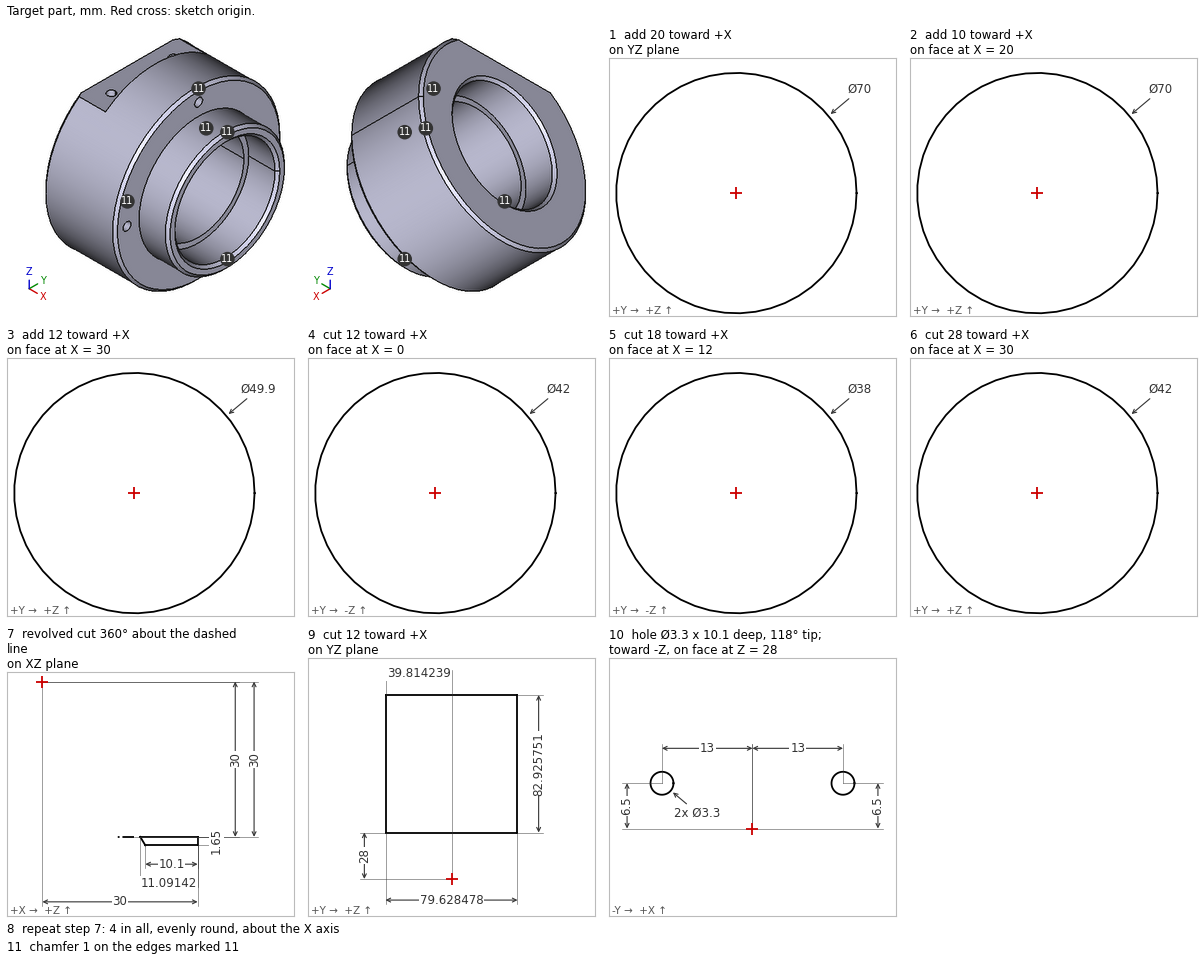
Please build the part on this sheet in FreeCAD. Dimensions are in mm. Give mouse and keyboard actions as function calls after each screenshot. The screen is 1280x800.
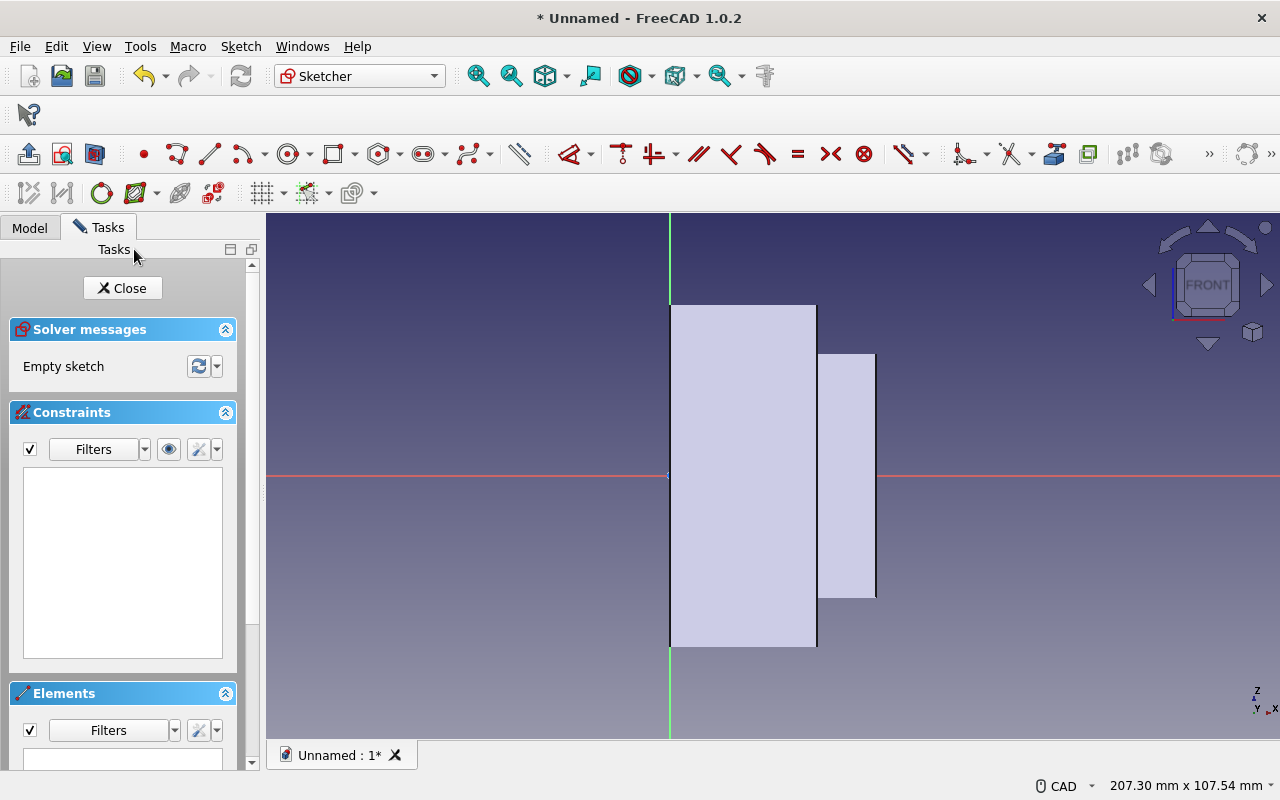
key(q)
key(s)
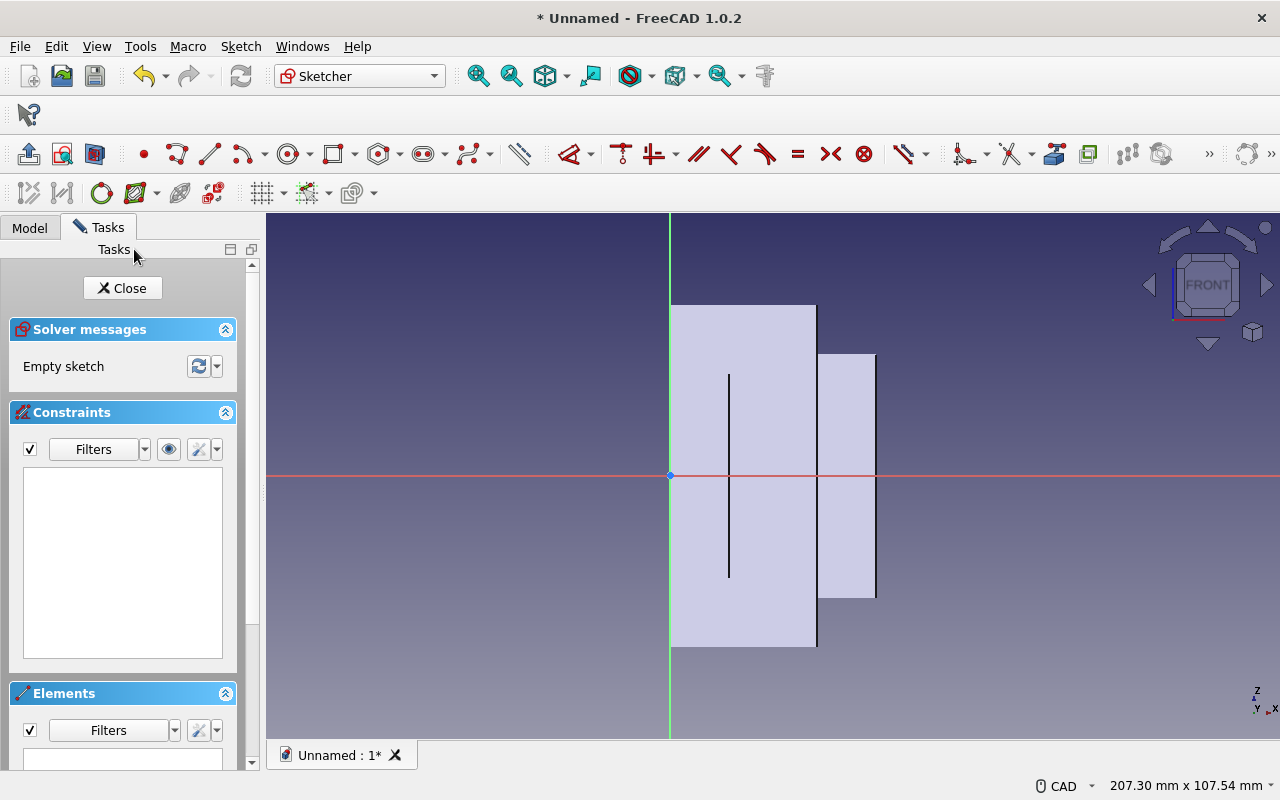
scroll(776, 617, up, 4)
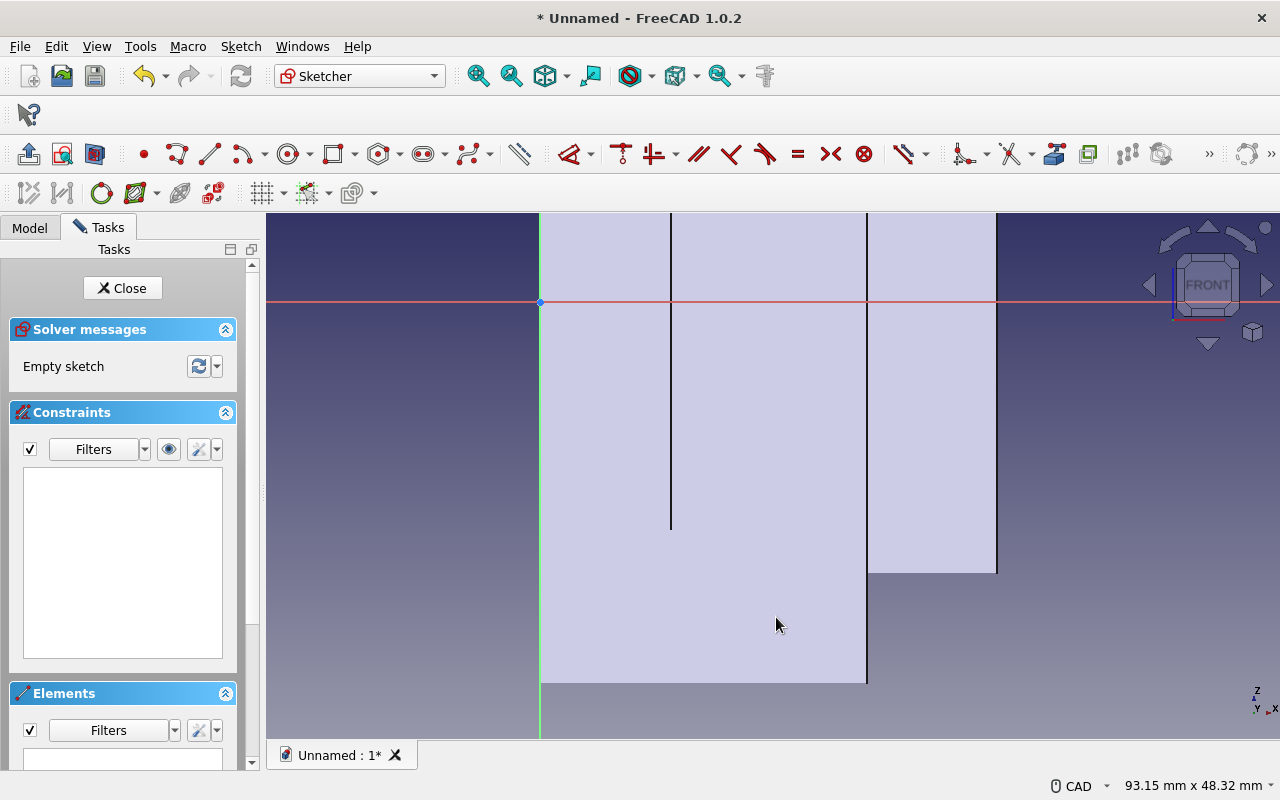
click(177, 154)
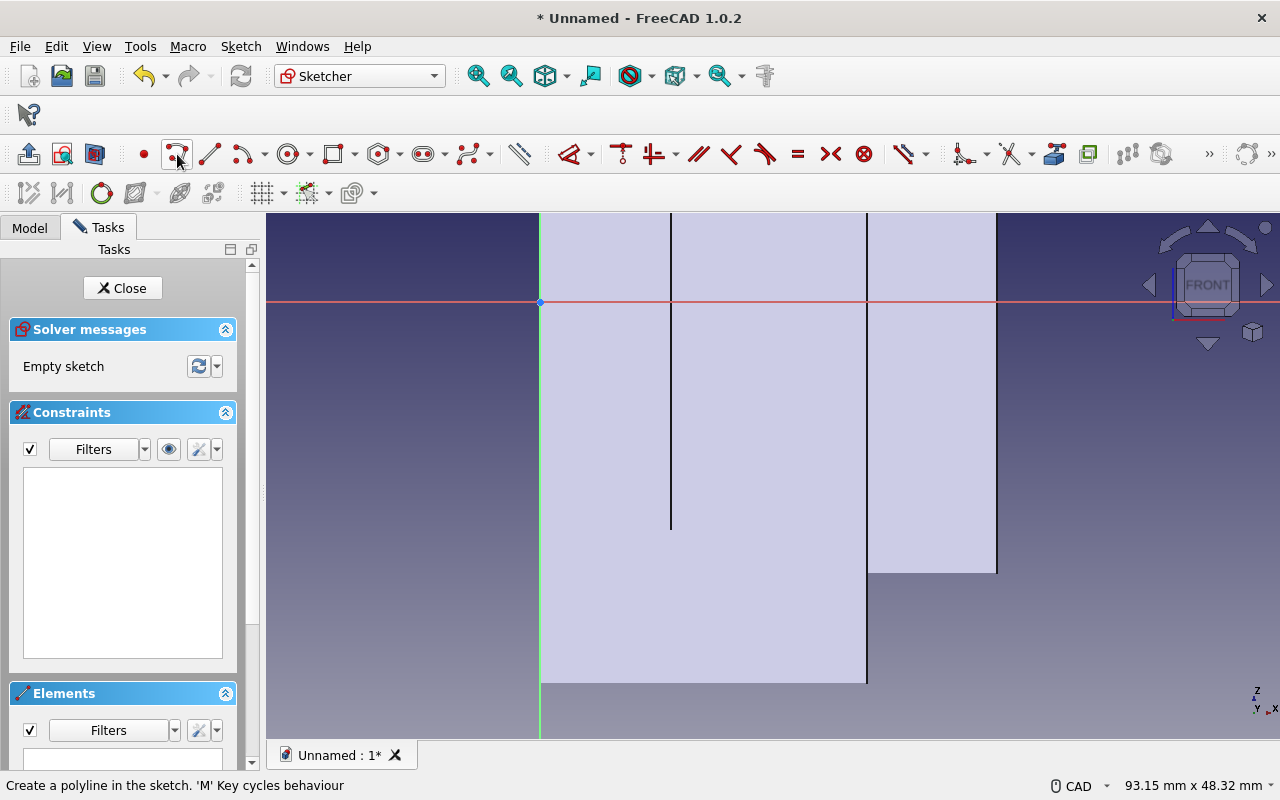
click(746, 629)
click(867, 629)
click(867, 647)
click(757, 647)
click(746, 630)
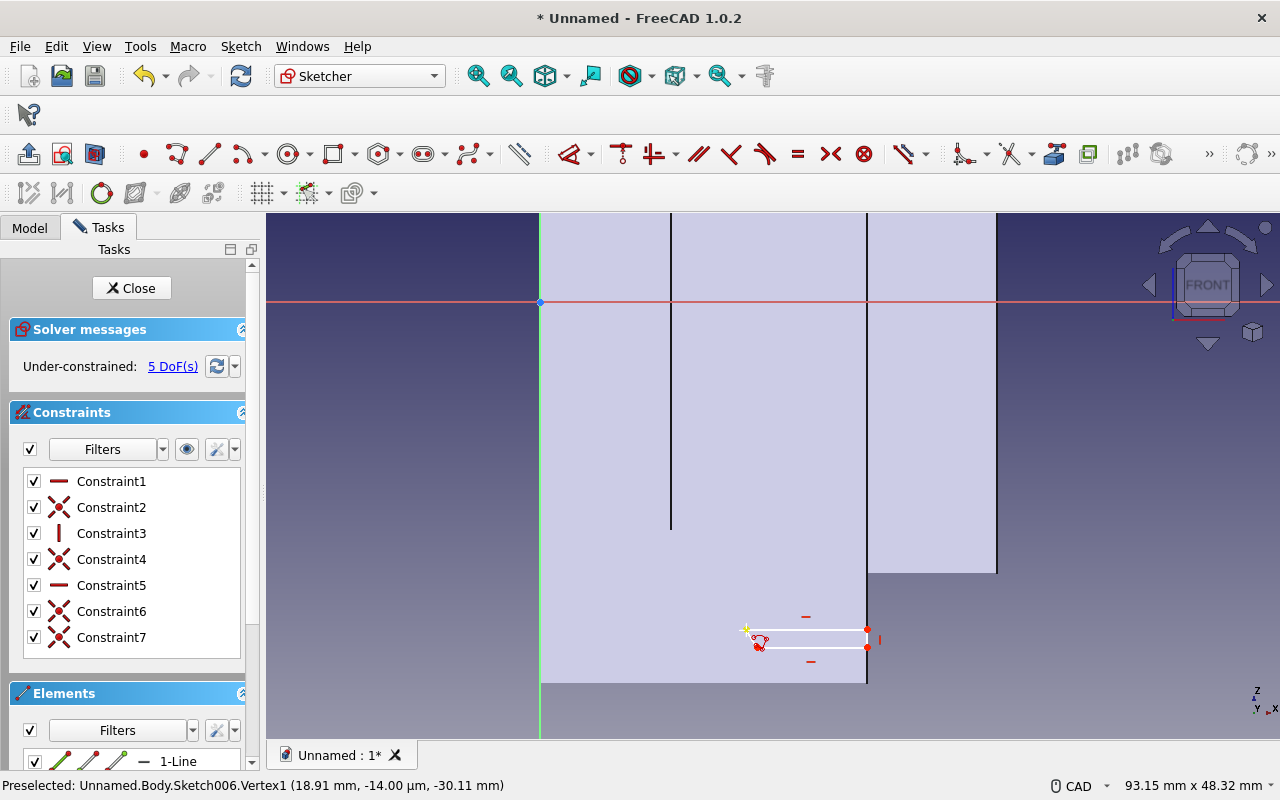
click(210, 154)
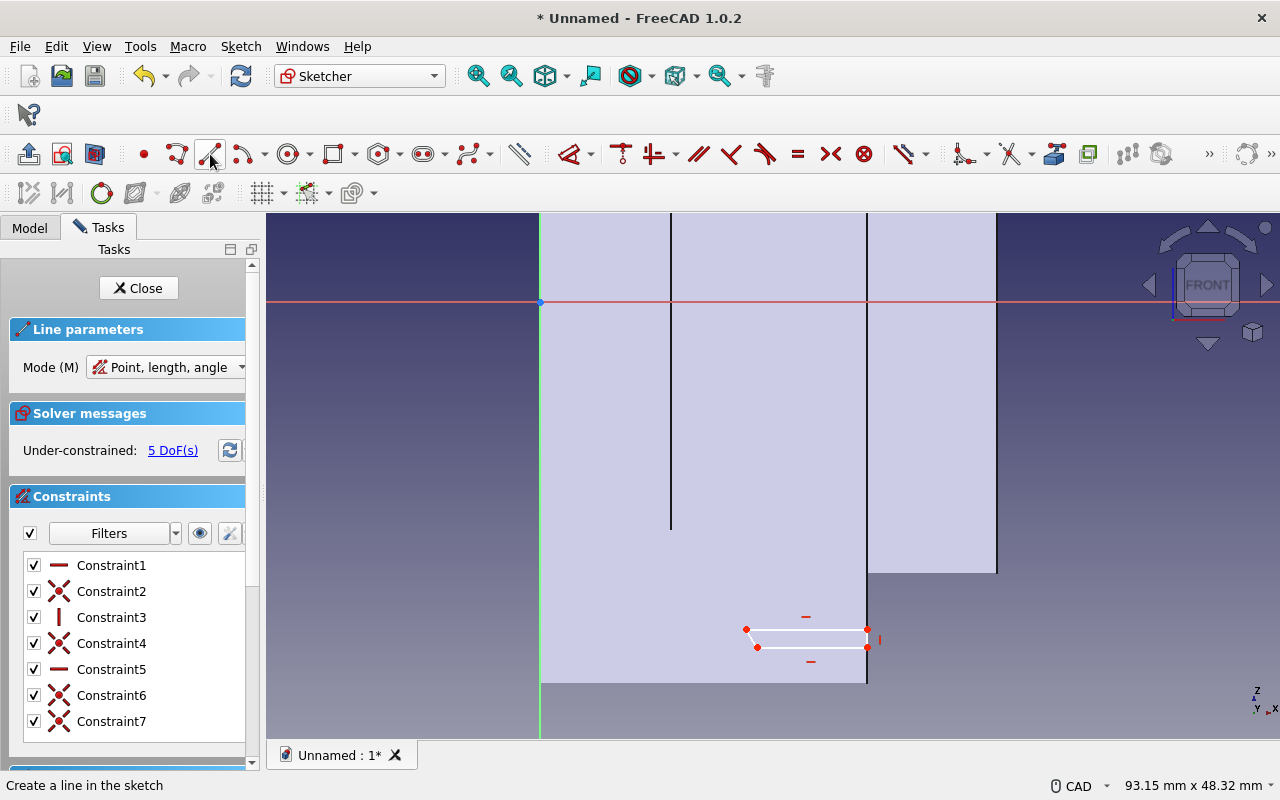
scroll(734, 629, up, 2)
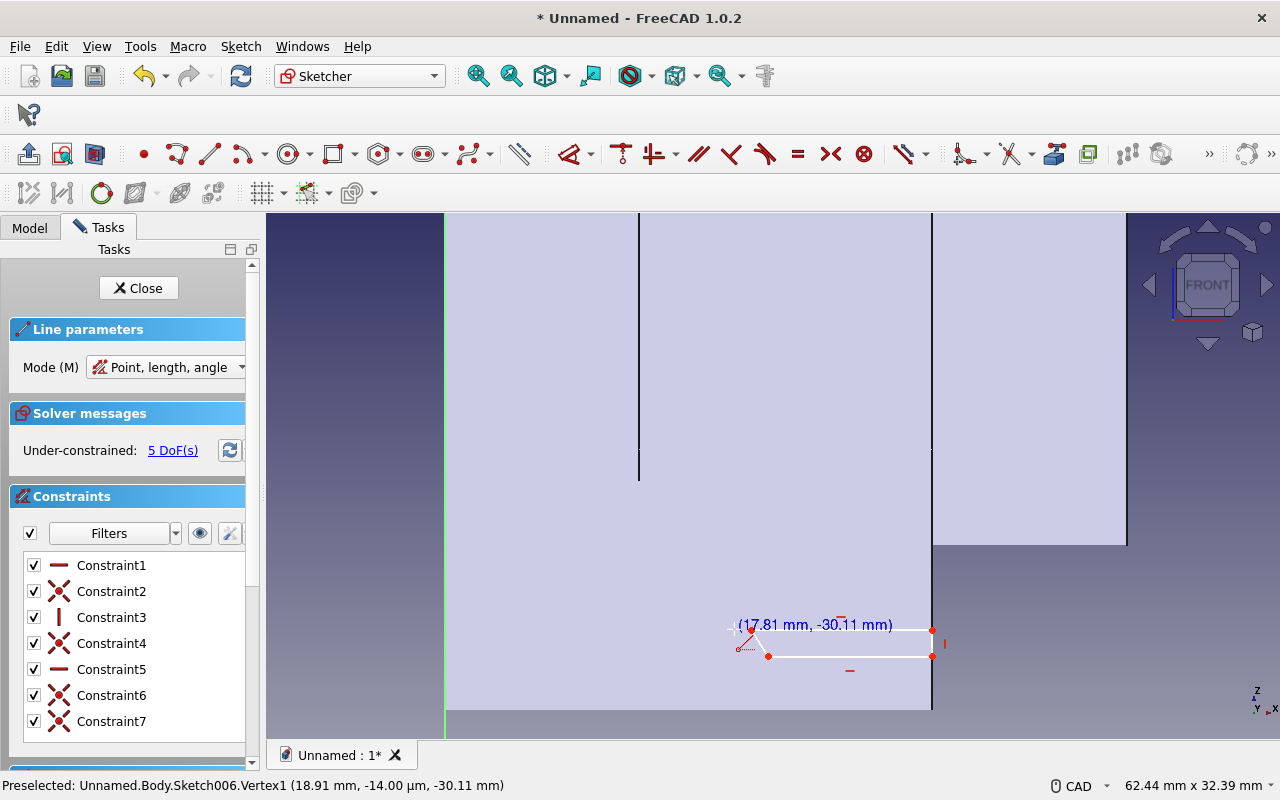
click(734, 628)
click(680, 628)
key(Escape)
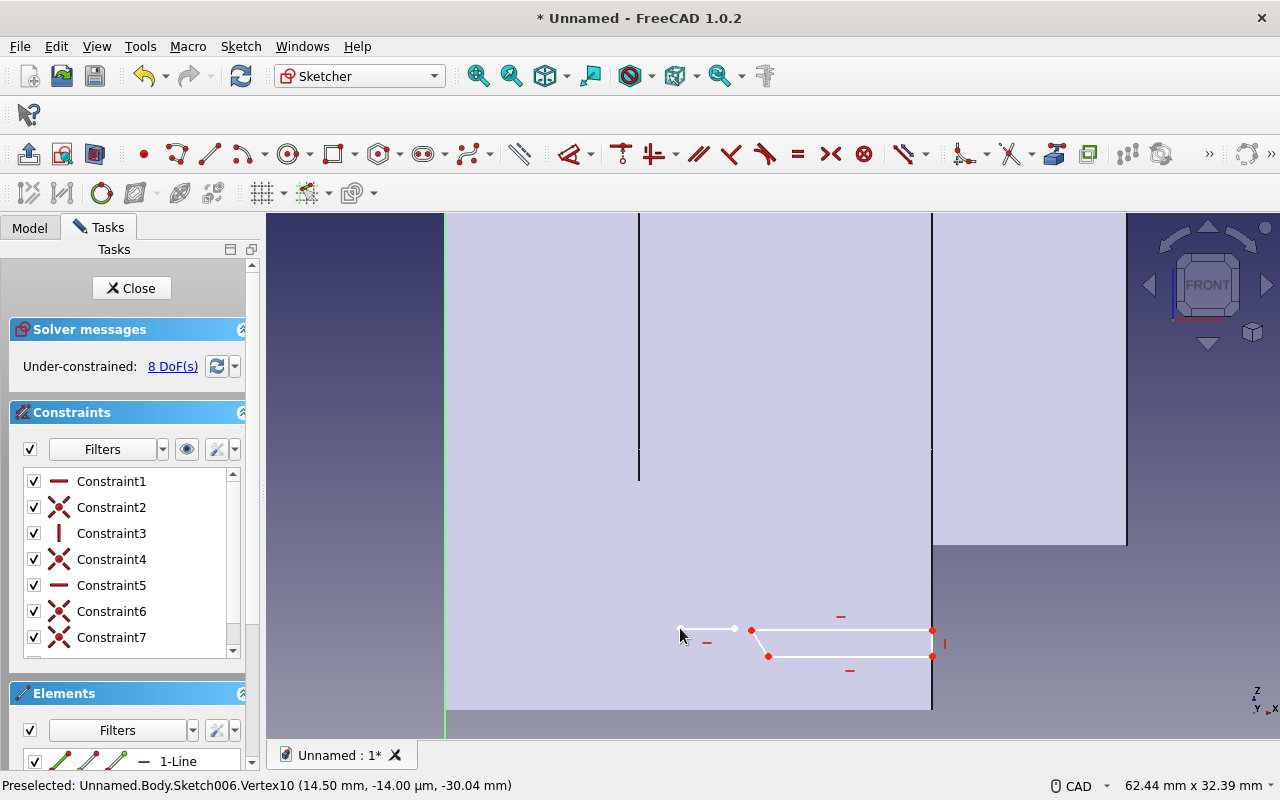
click(718, 629)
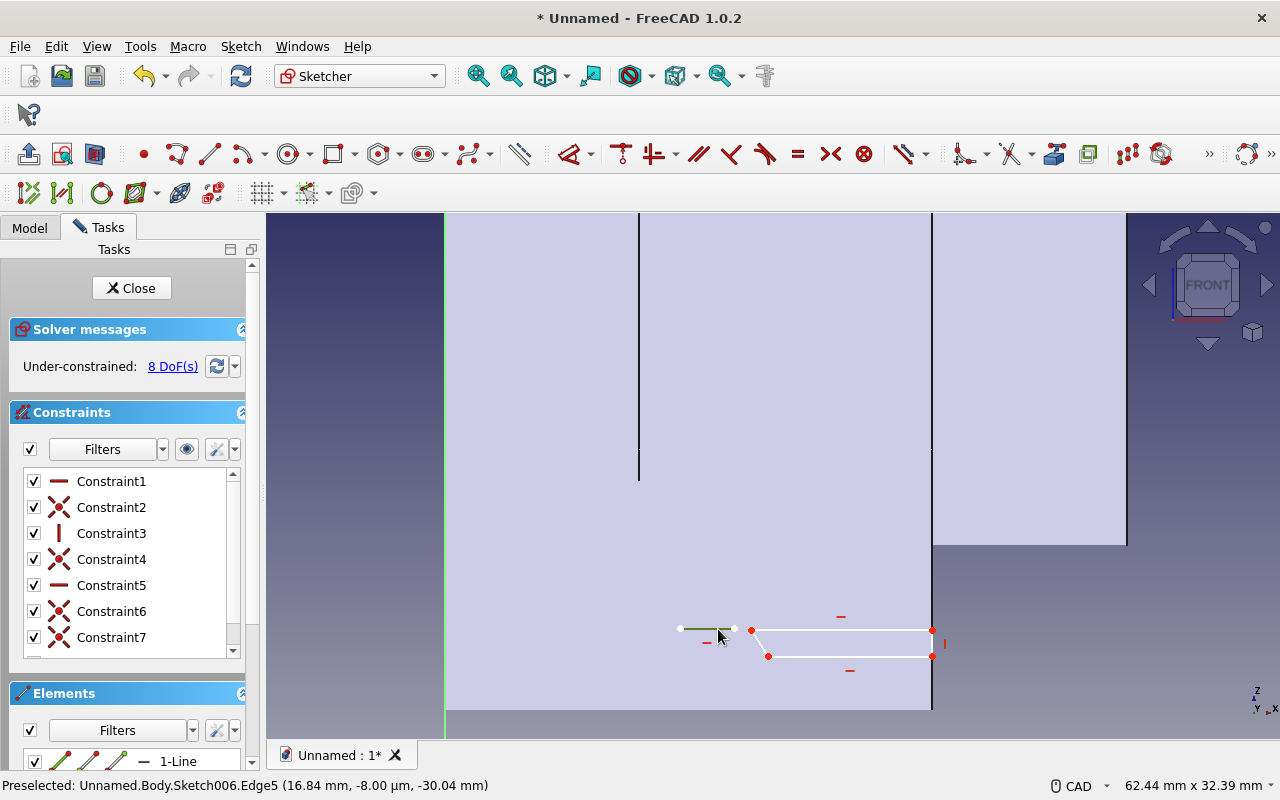
click(520, 154)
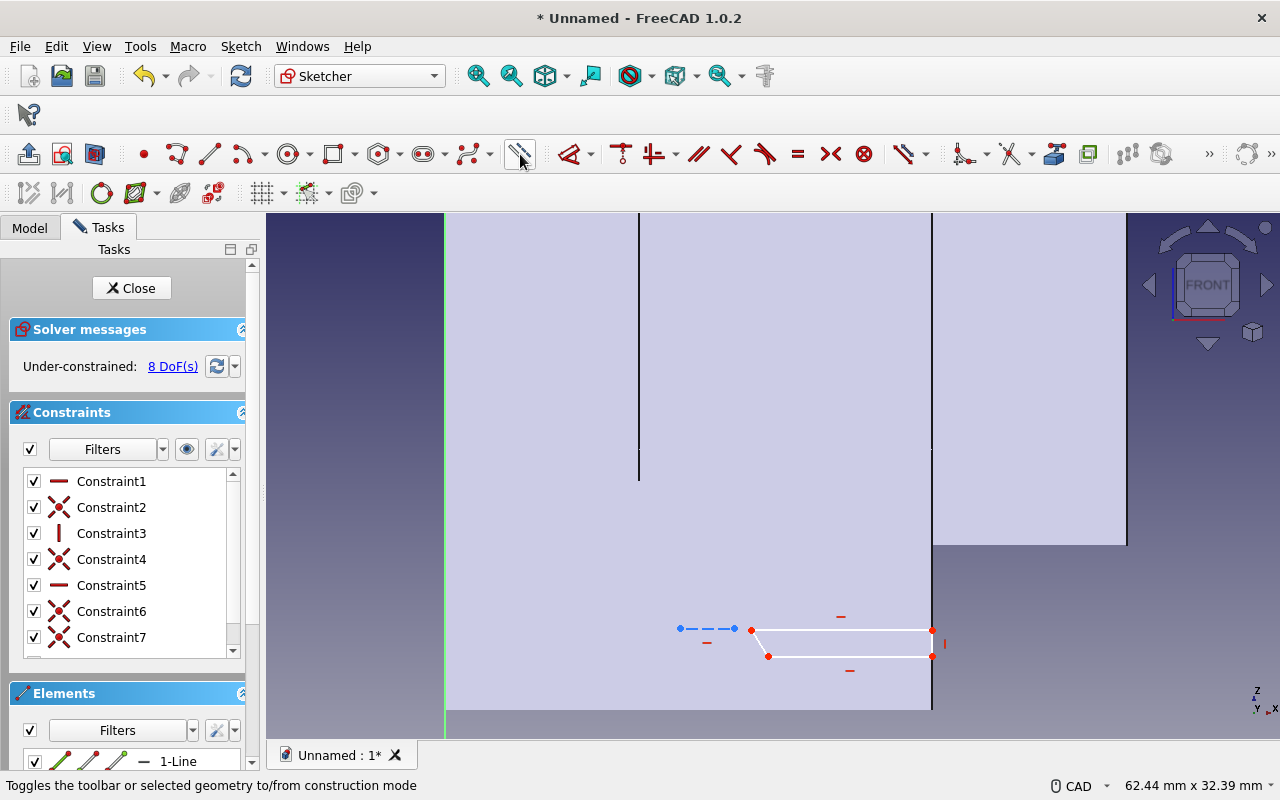
click(568, 154)